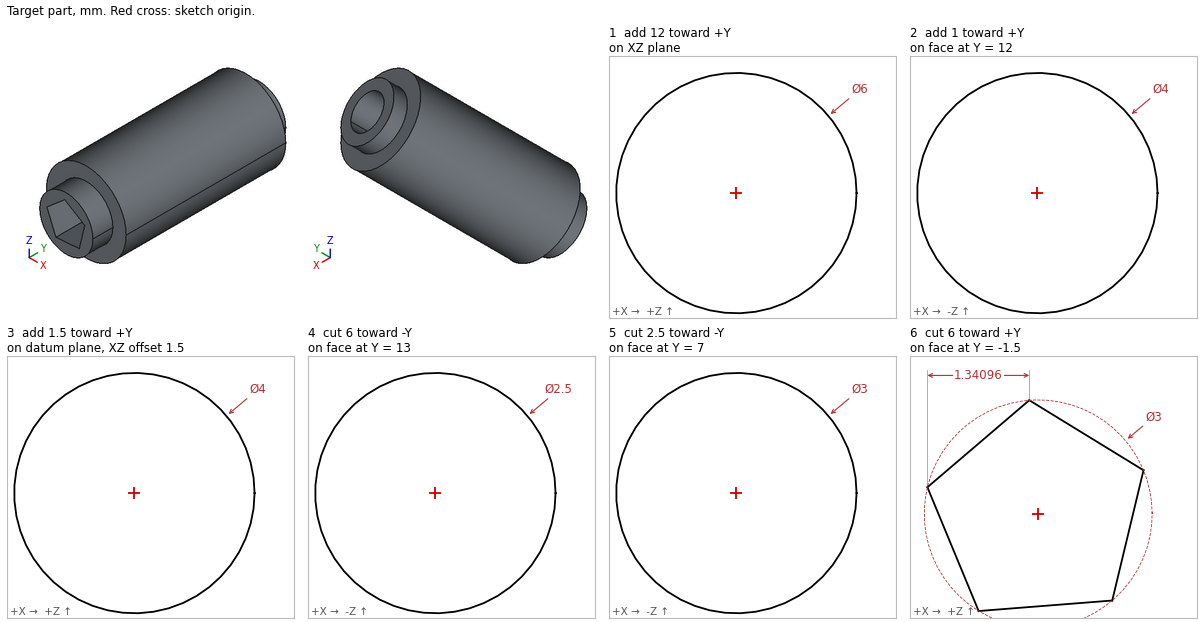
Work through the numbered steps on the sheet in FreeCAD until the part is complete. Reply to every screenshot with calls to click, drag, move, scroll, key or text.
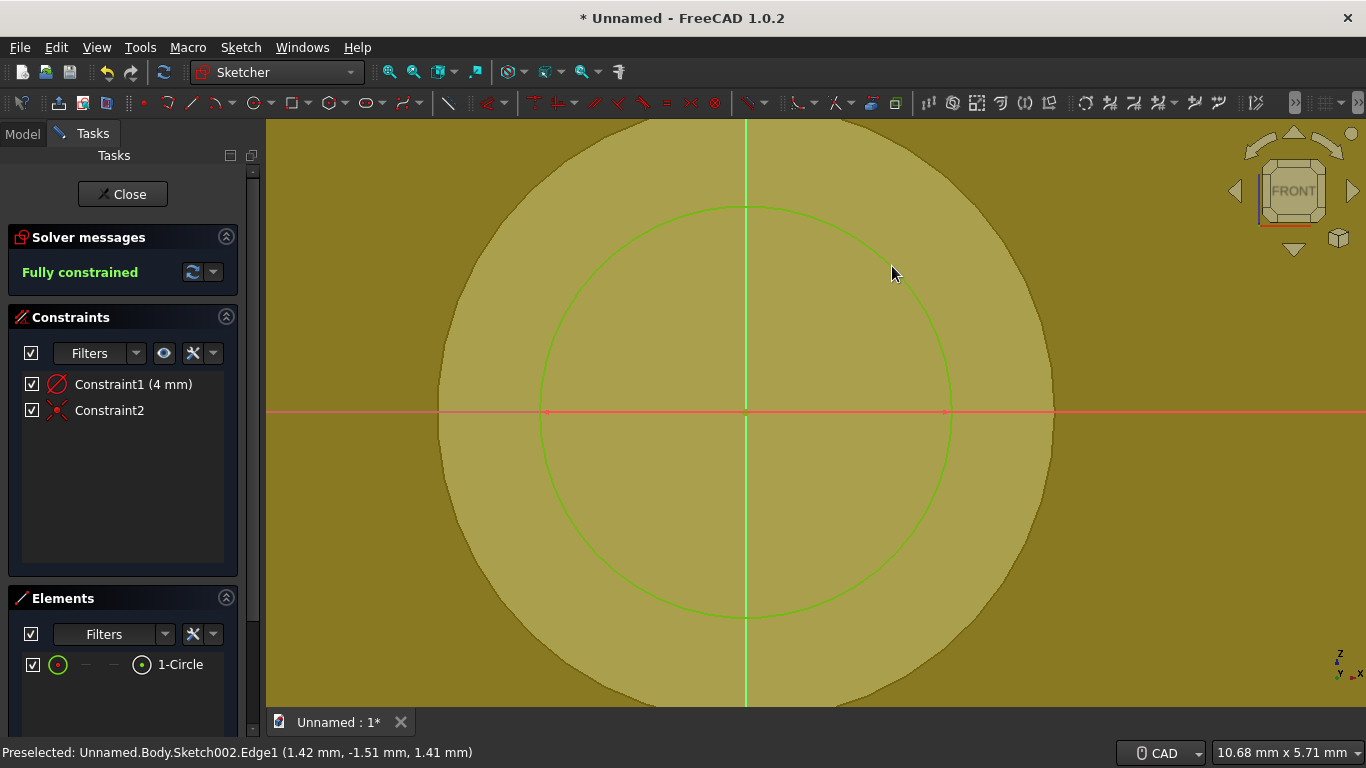
click(123, 194)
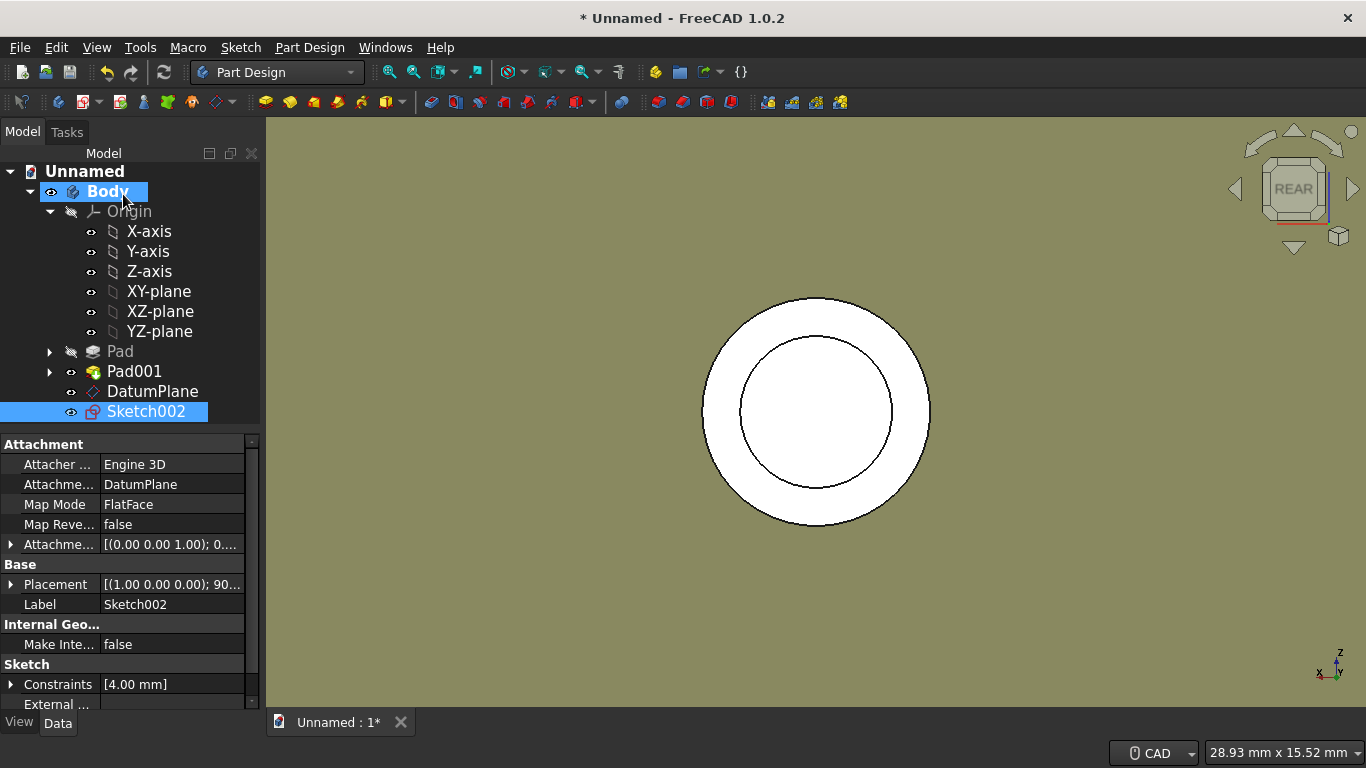
click(266, 102)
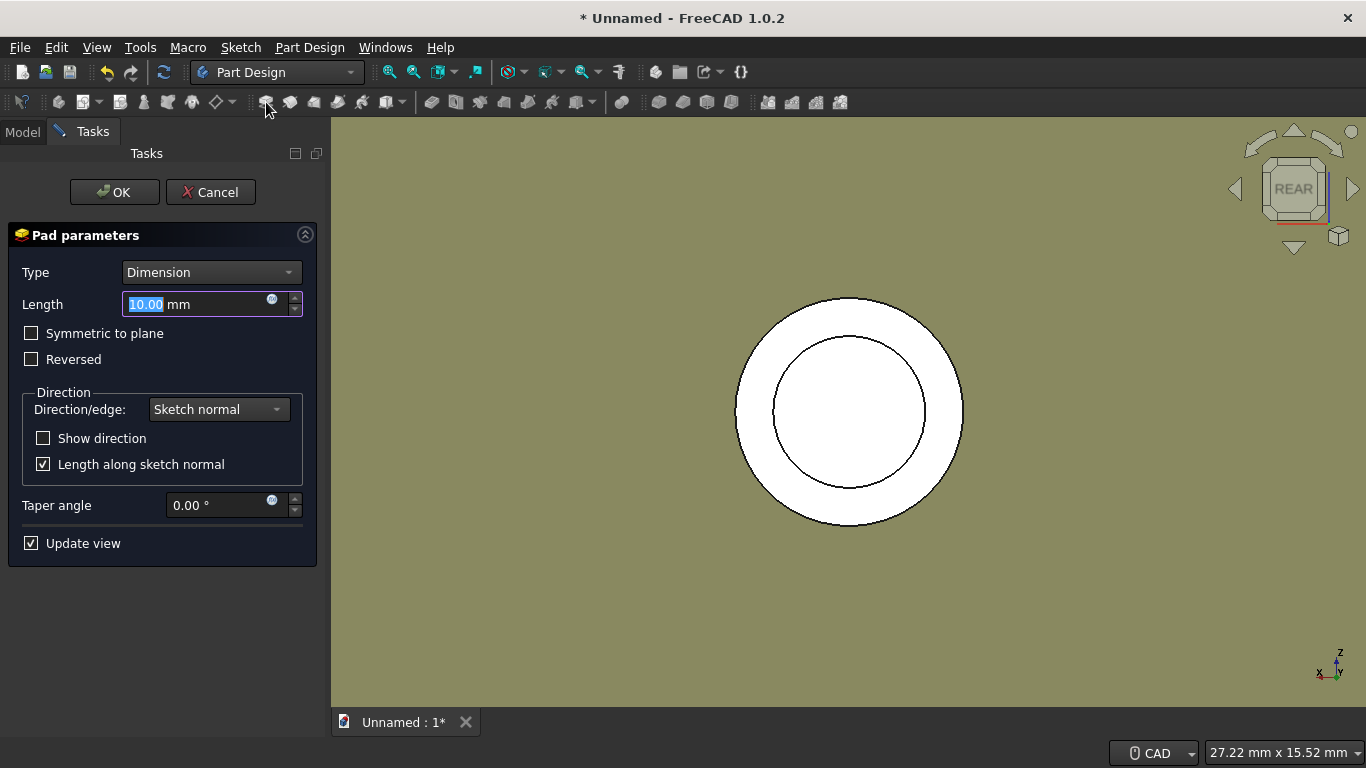
text(1.5)
key(Tab)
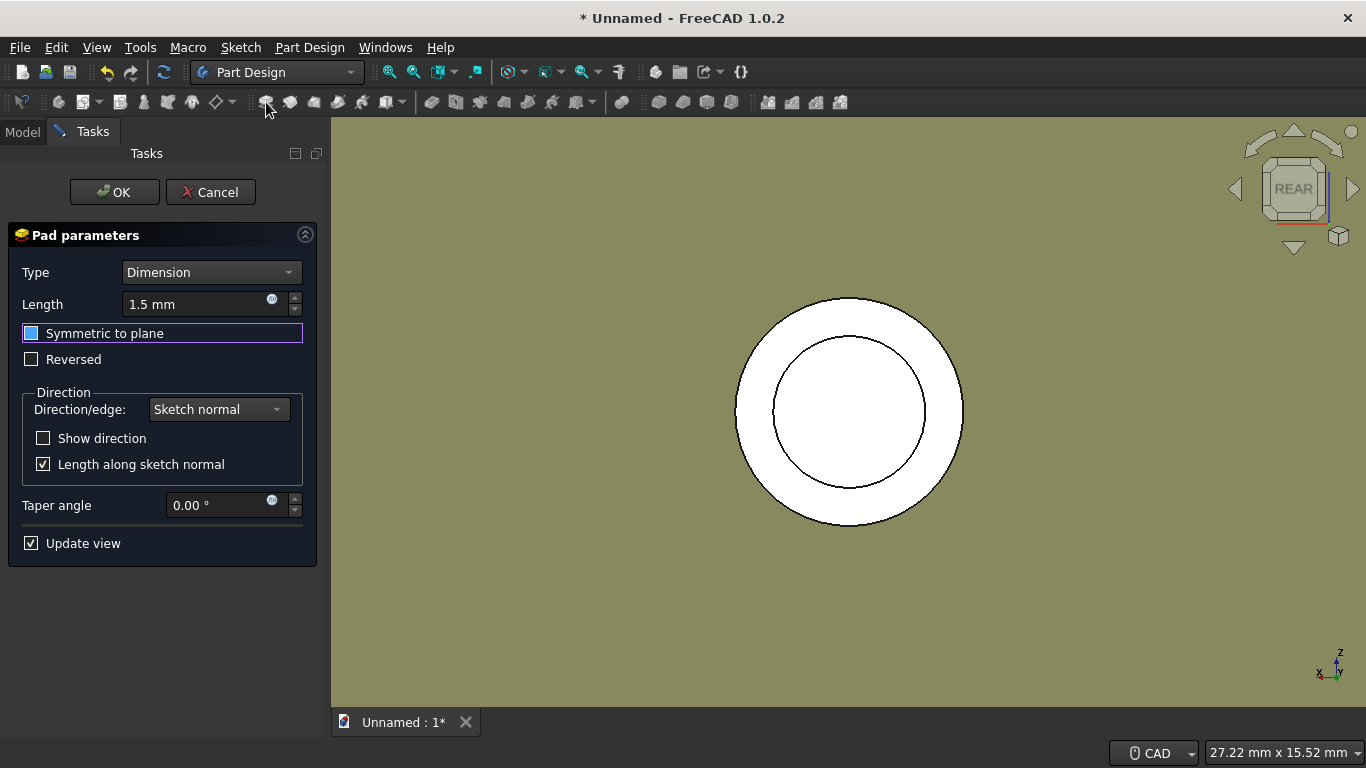
click(30, 359)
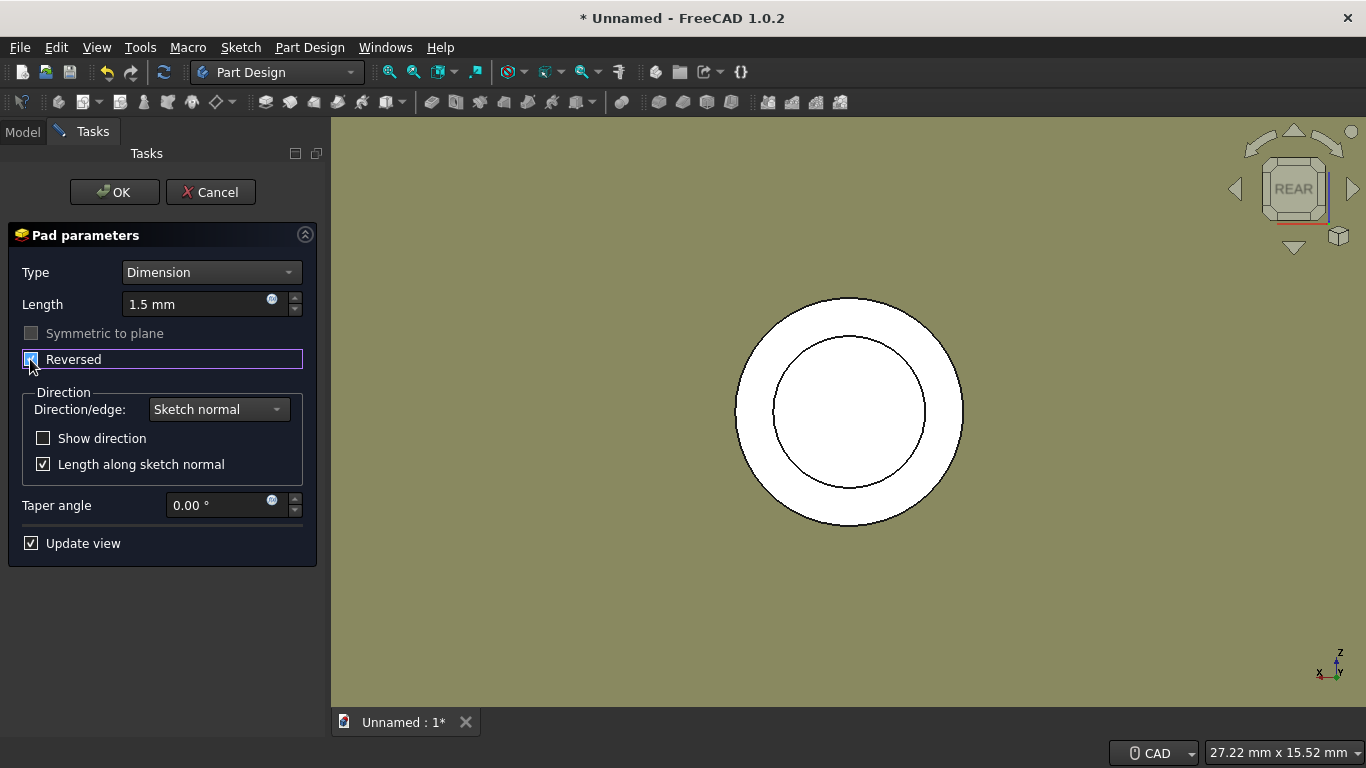
click(115, 192)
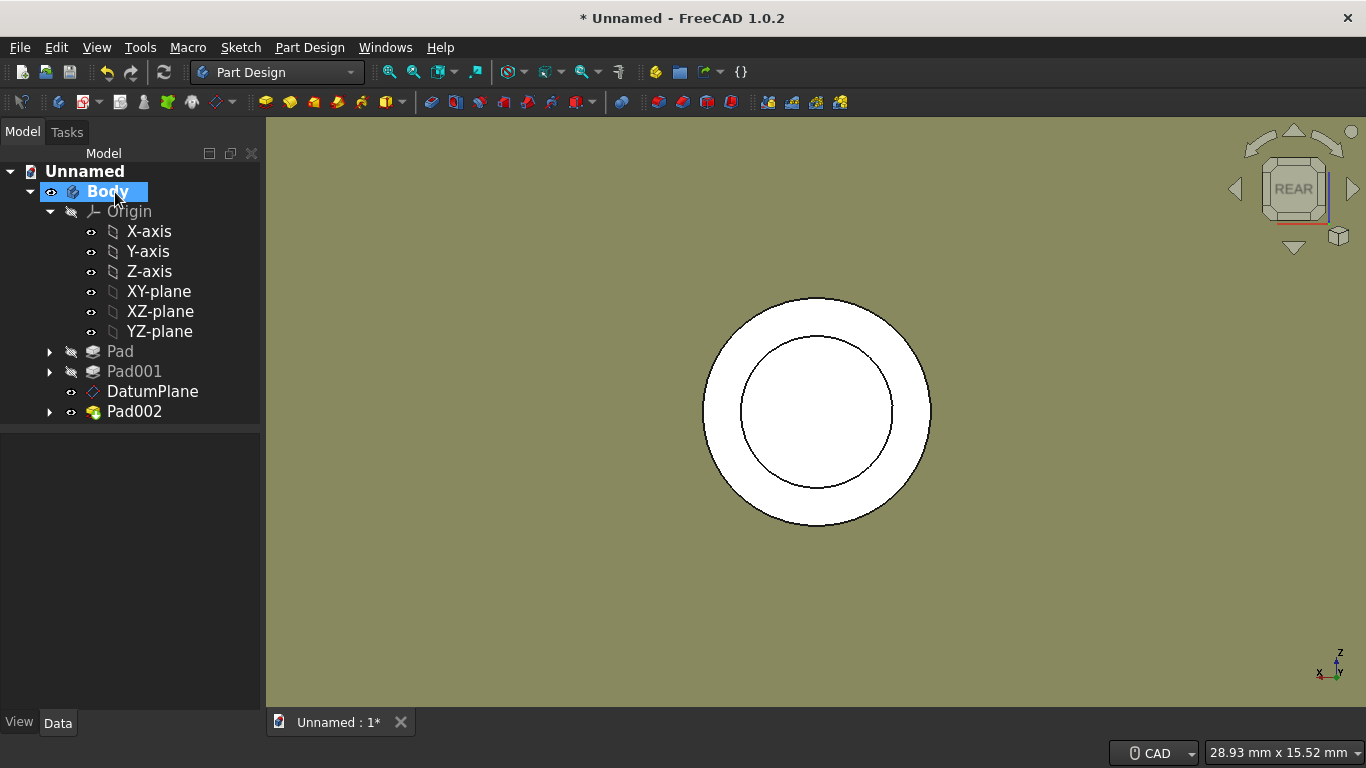
click(116, 392)
key(space)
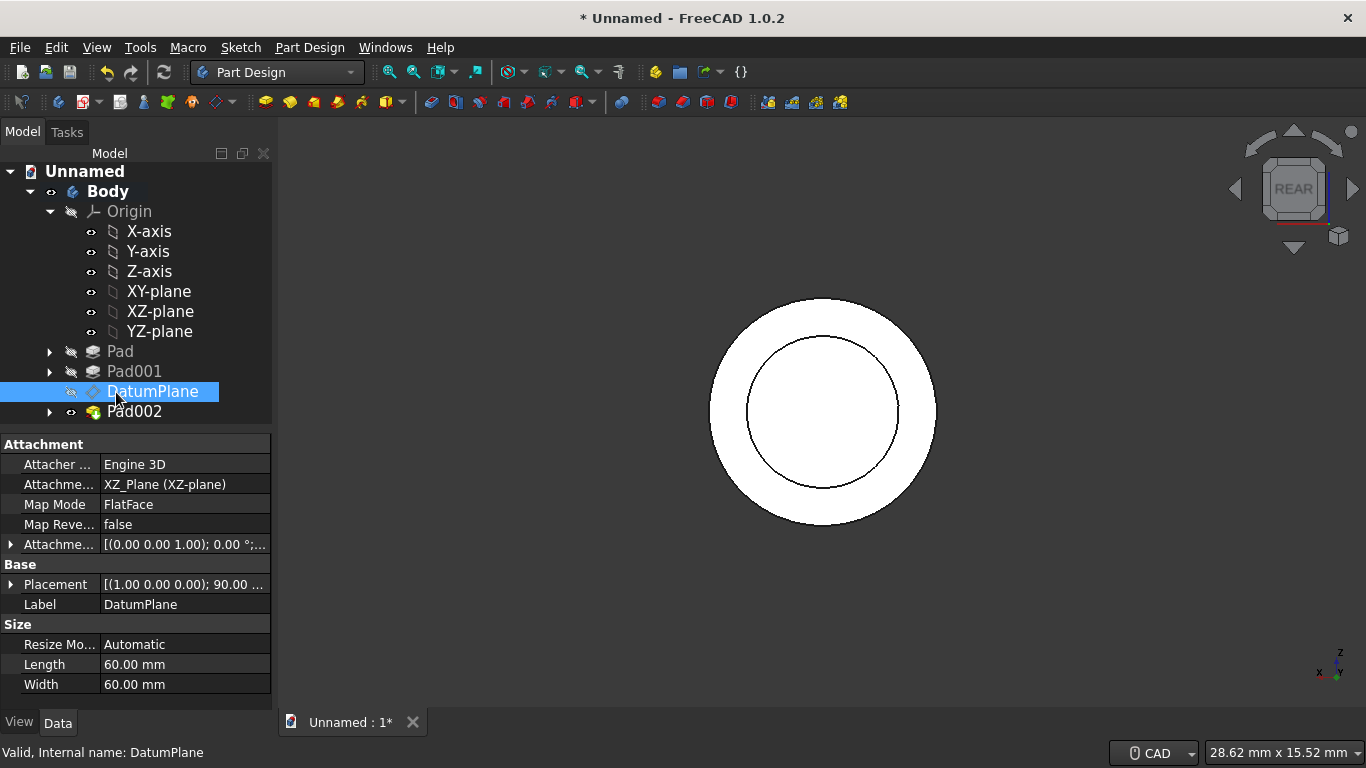
click(390, 72)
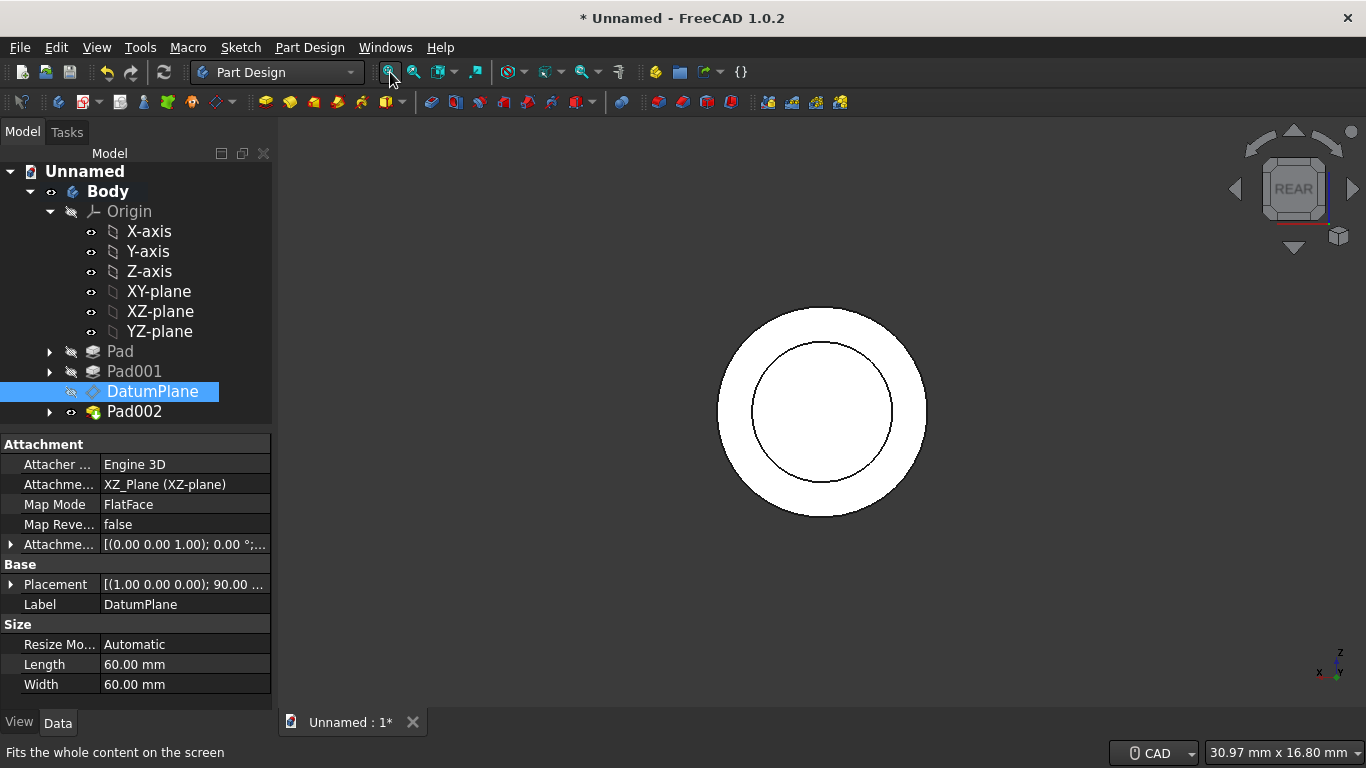
click(822, 411)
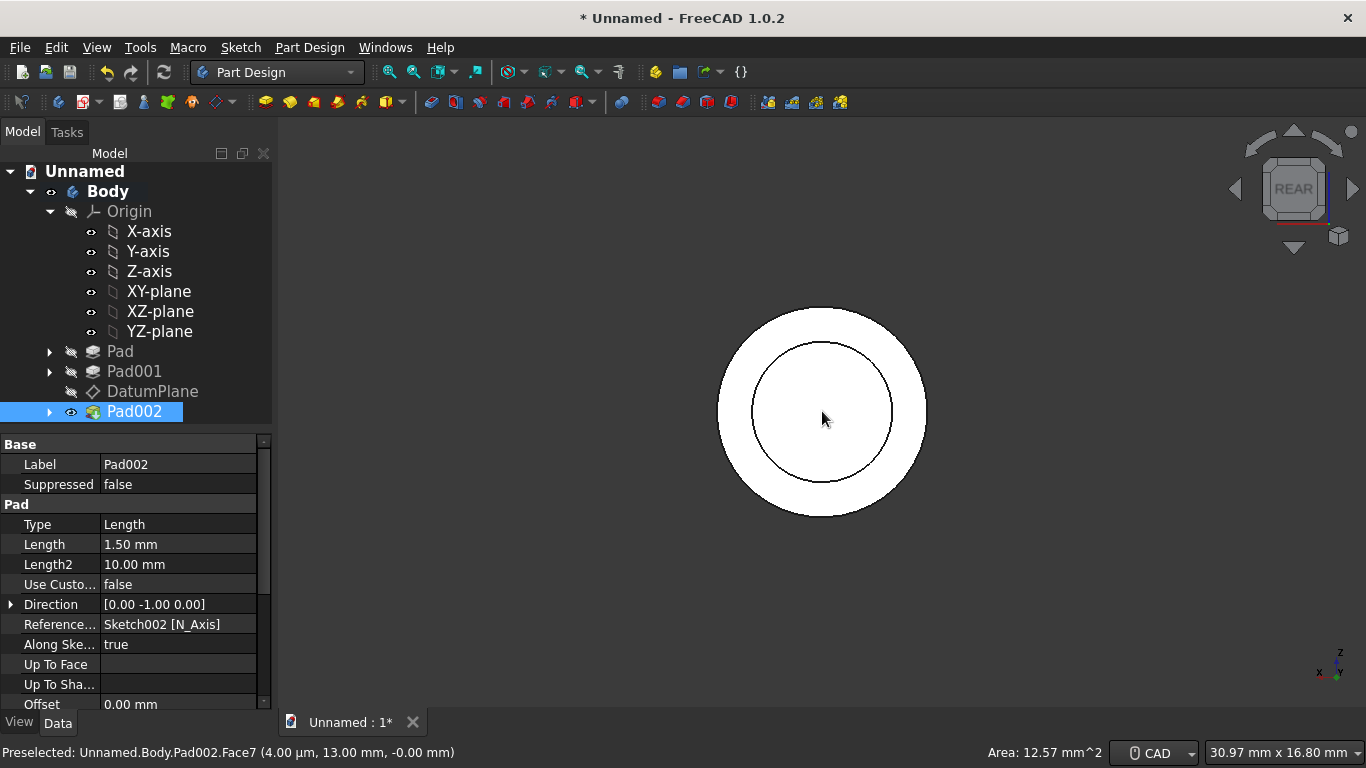
click(84, 102)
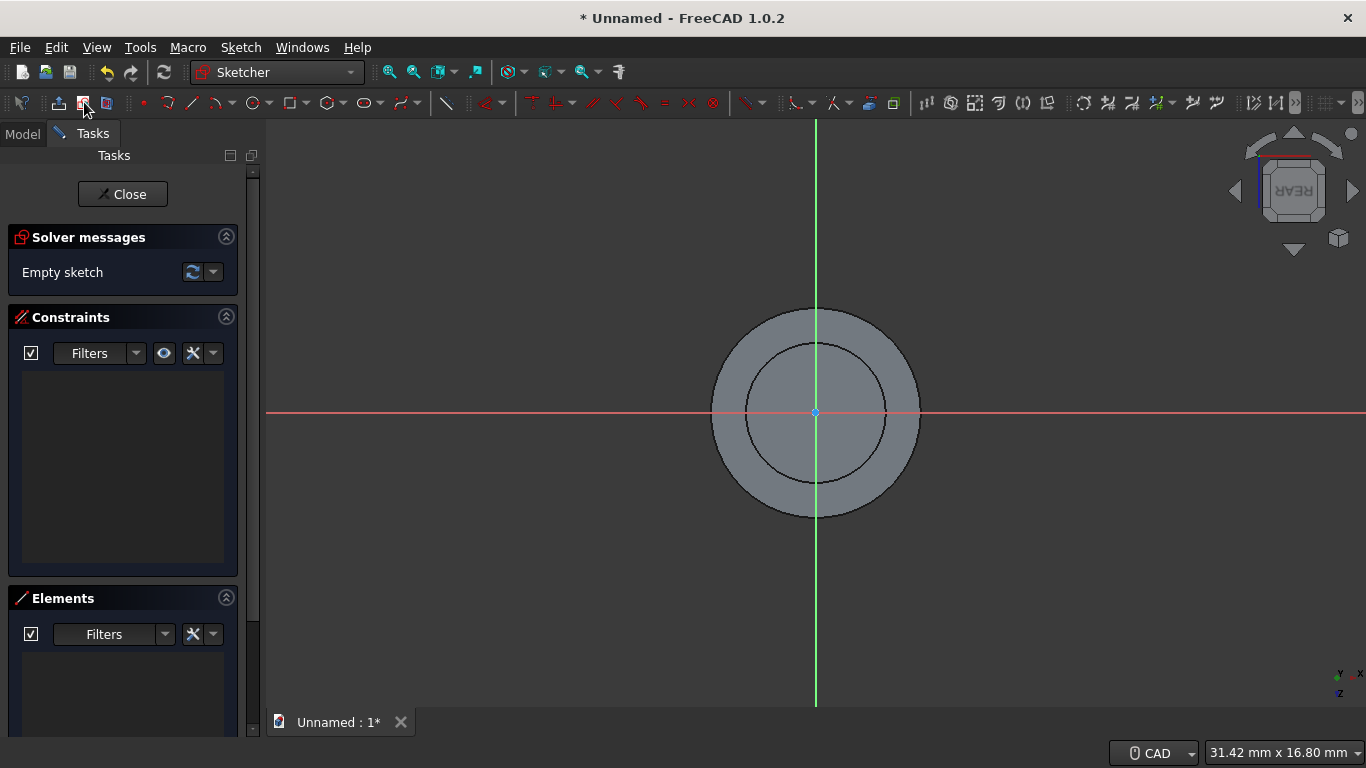
scroll(838, 413, up, 7)